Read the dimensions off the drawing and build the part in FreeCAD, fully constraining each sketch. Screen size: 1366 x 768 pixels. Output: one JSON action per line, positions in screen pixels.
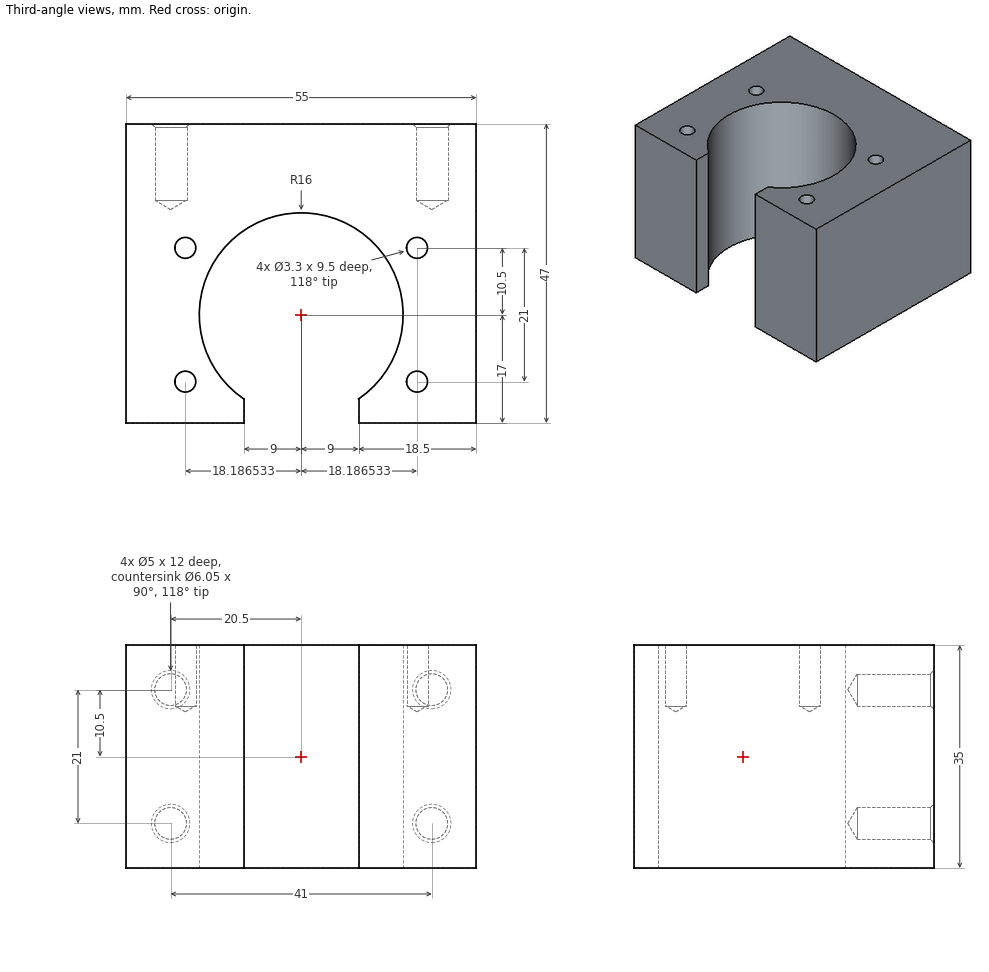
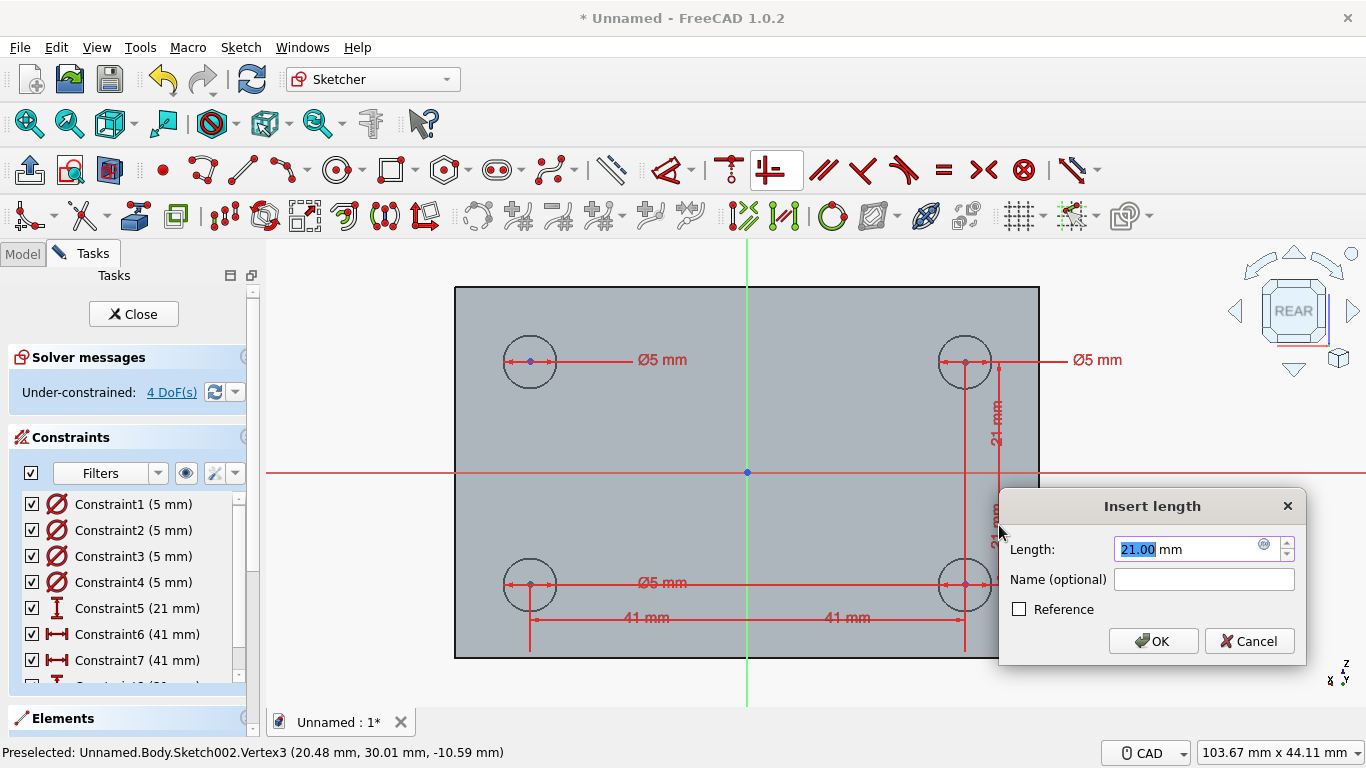
{"action": "type", "text": "21"}
{"action": "key", "text": "Return"}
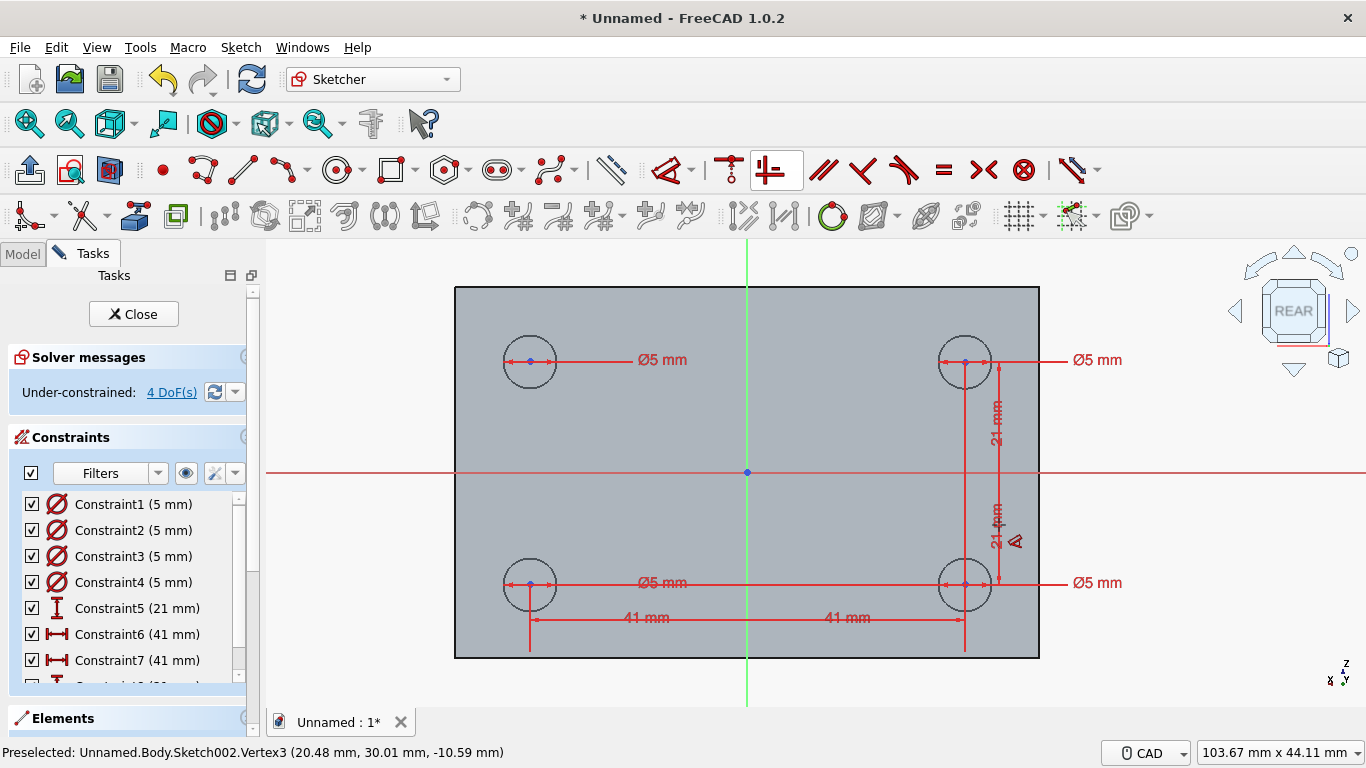
{"action": "left_click", "coordinate": [965, 362]}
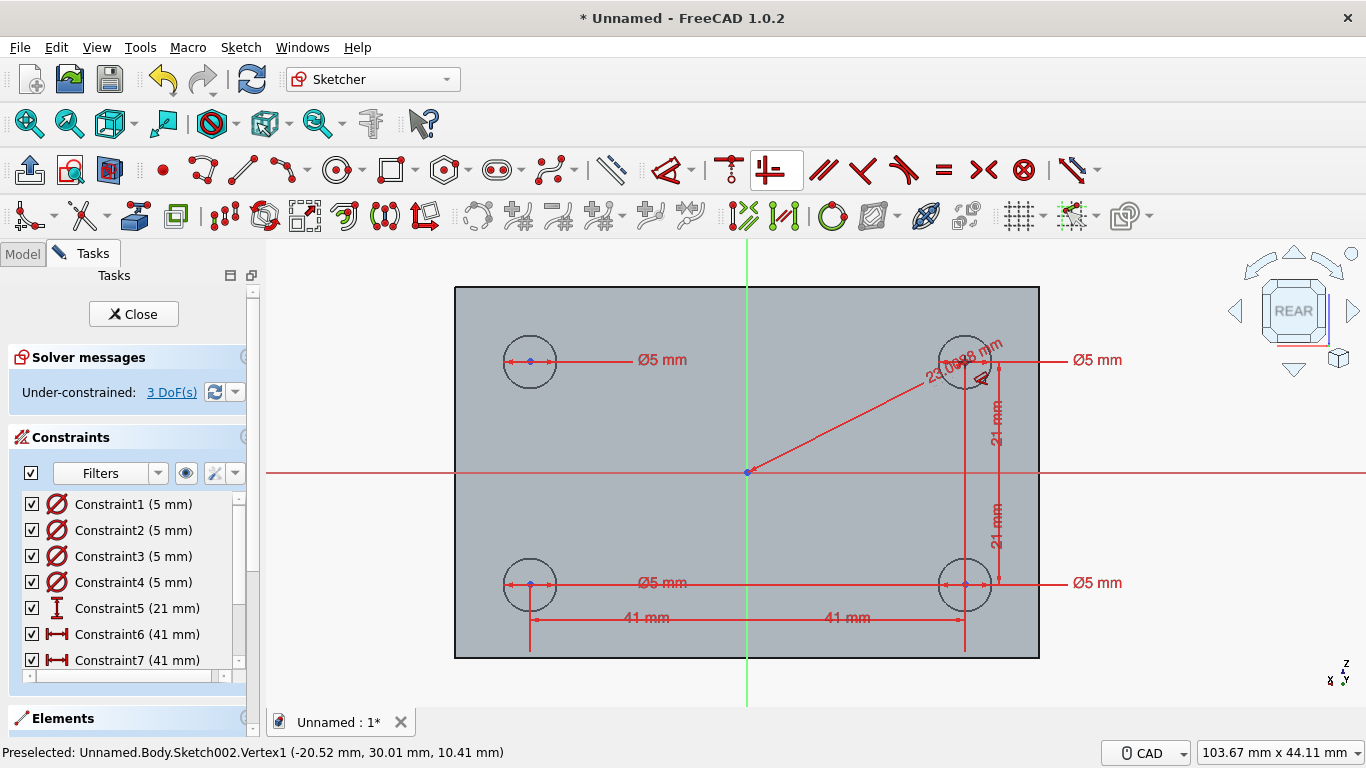
{"action": "left_click", "coordinate": [530, 362]}
{"action": "left_click", "coordinate": [647, 328]}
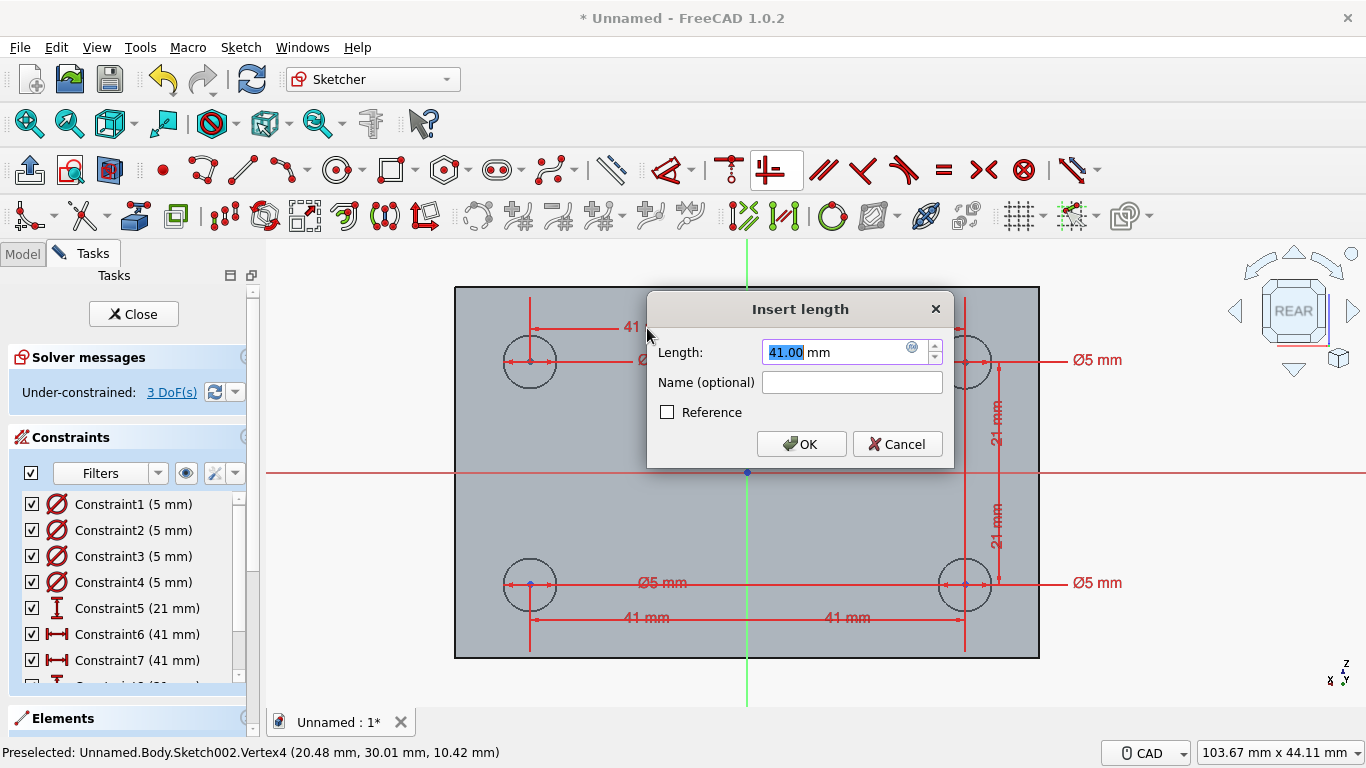
{"action": "type", "text": "41"}
{"action": "key", "text": "Return"}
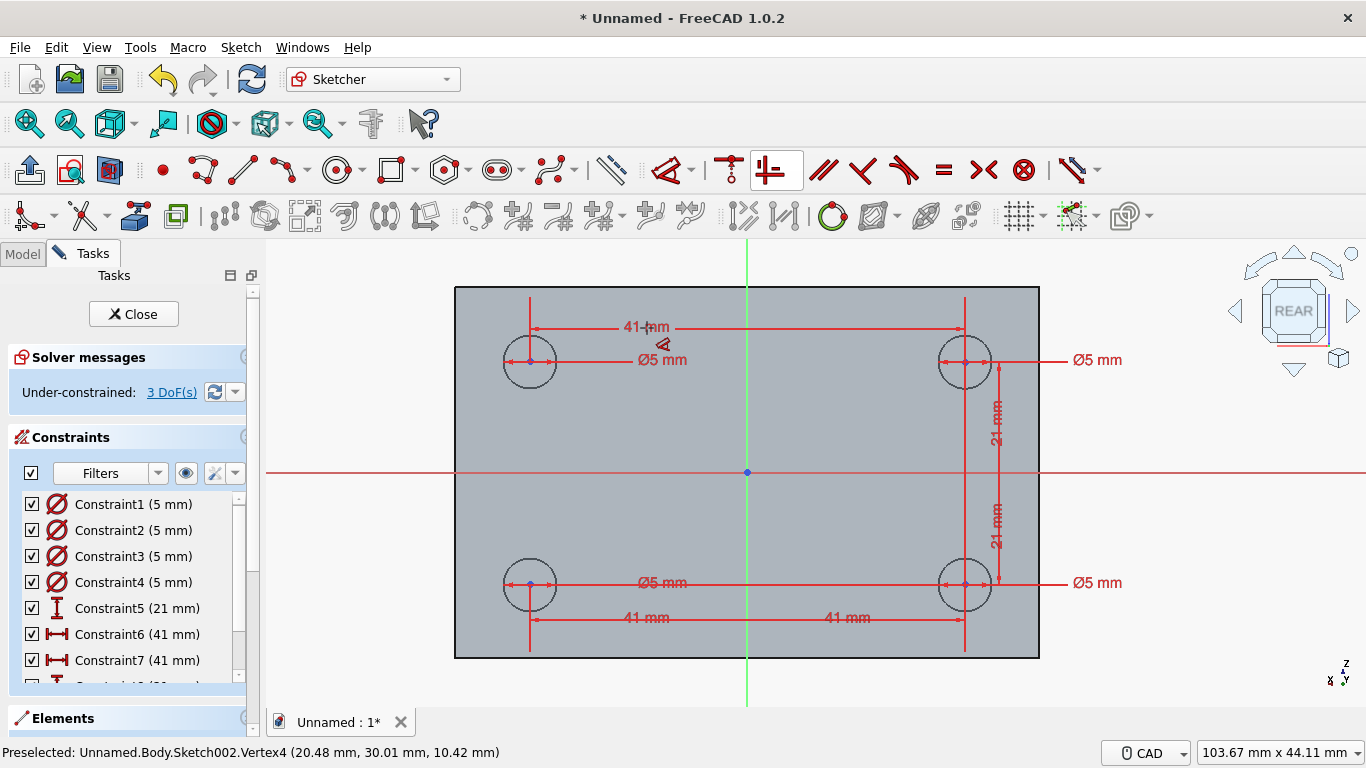
{"action": "left_click", "coordinate": [530, 585]}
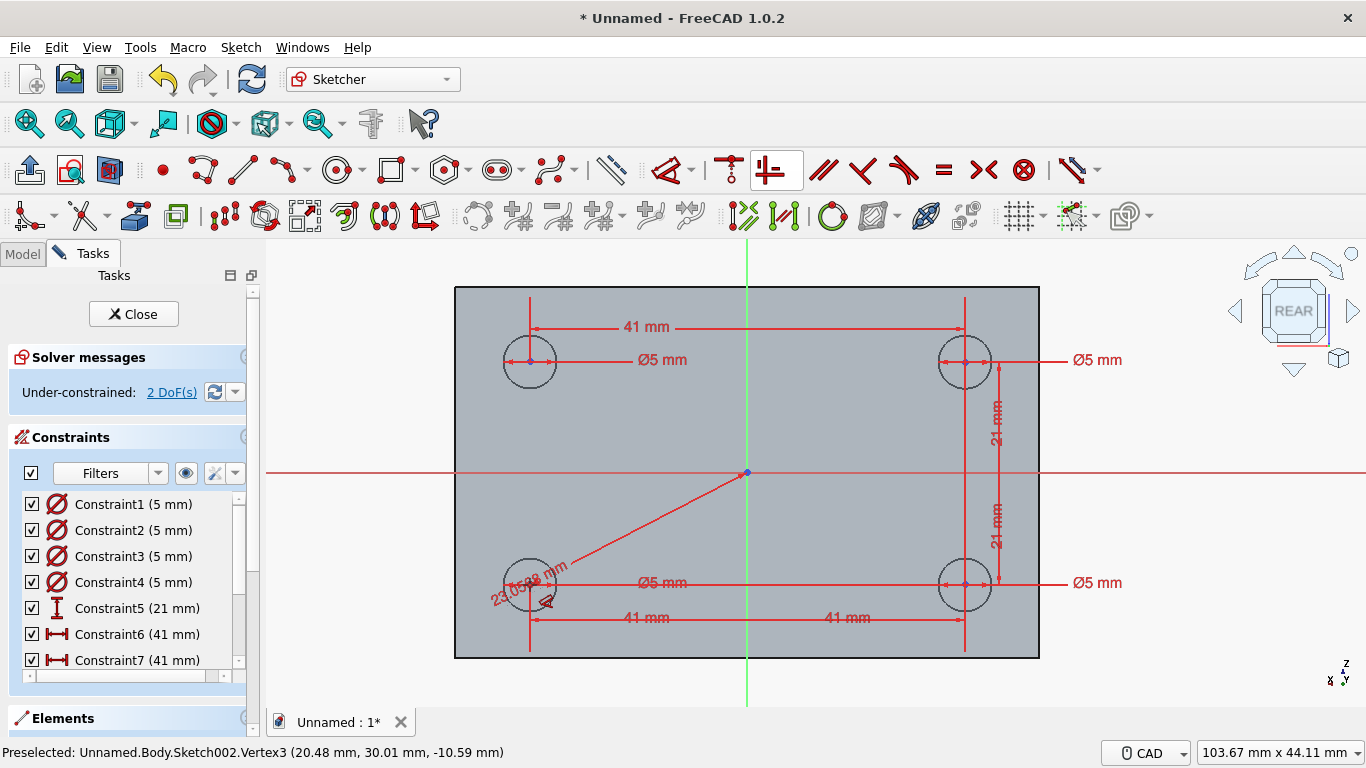
{"action": "left_click", "coordinate": [530, 362]}
{"action": "left_click", "coordinate": [496, 422]}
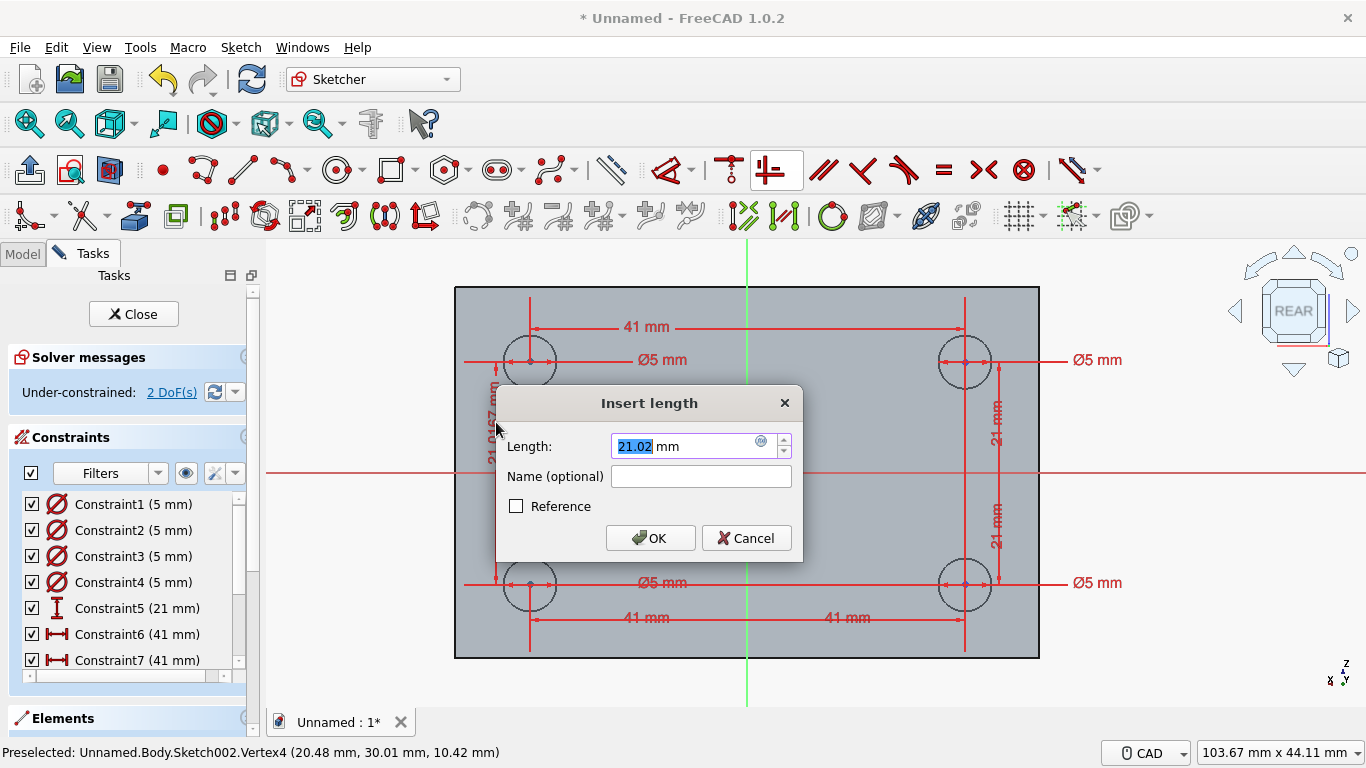
{"action": "type", "text": "21"}
{"action": "key", "text": "Return"}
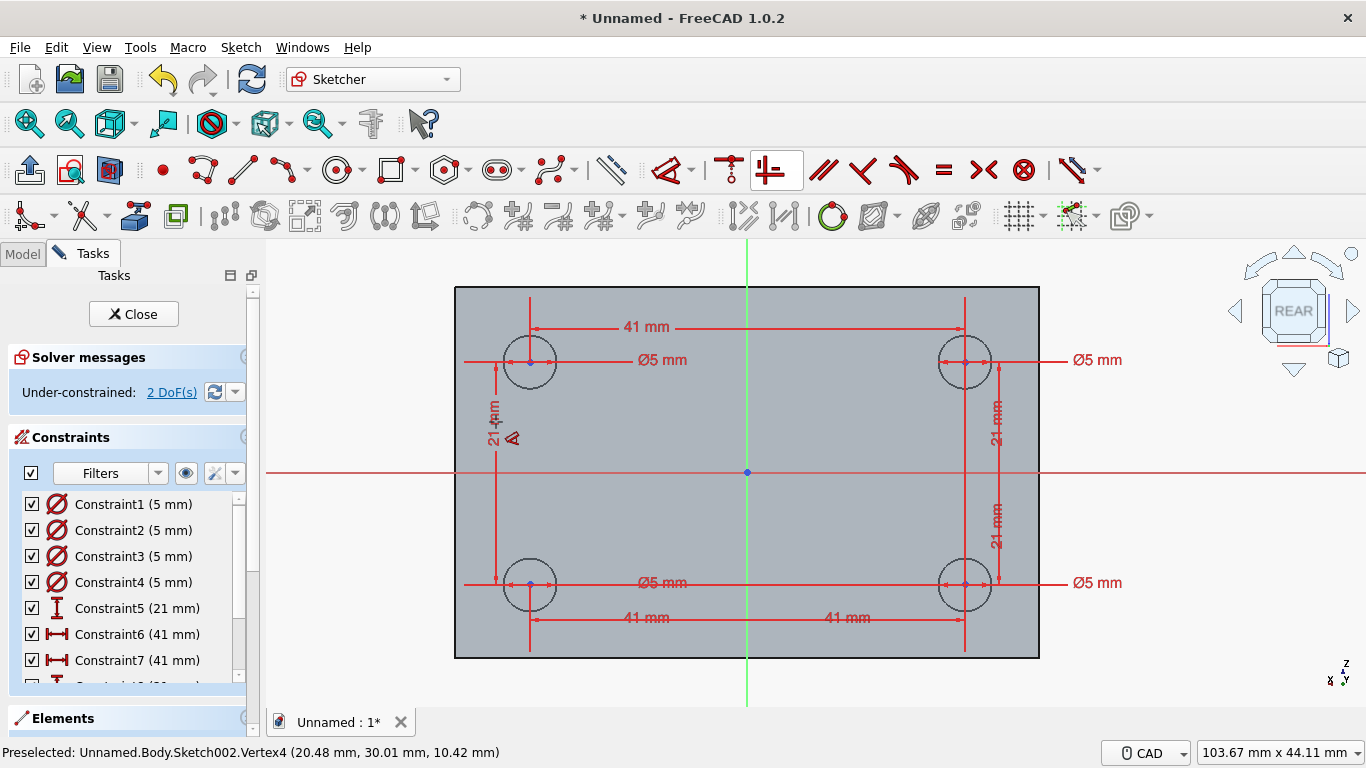
{"action": "left_click", "coordinate": [965, 362]}
{"action": "left_click", "coordinate": [856, 328]}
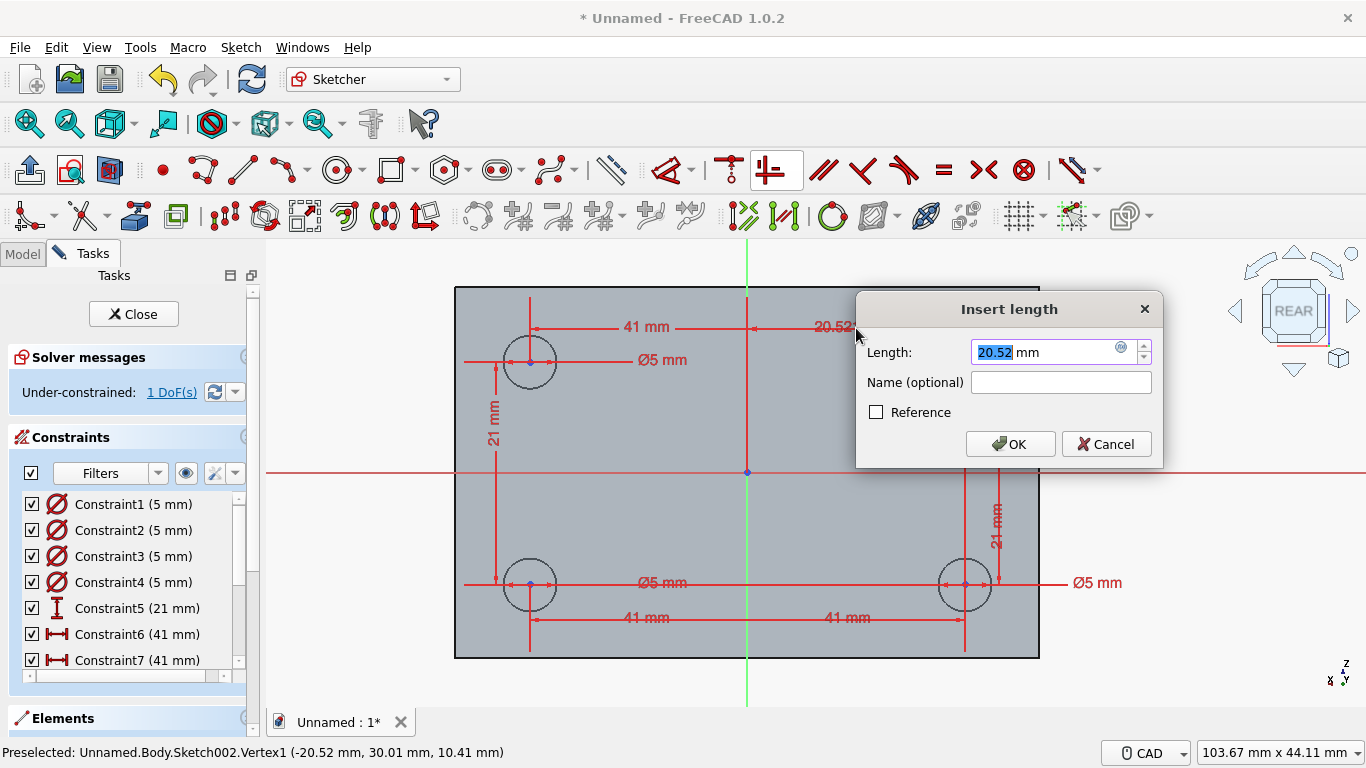
{"action": "type", "text": "20.5"}
{"action": "key", "text": "Return"}